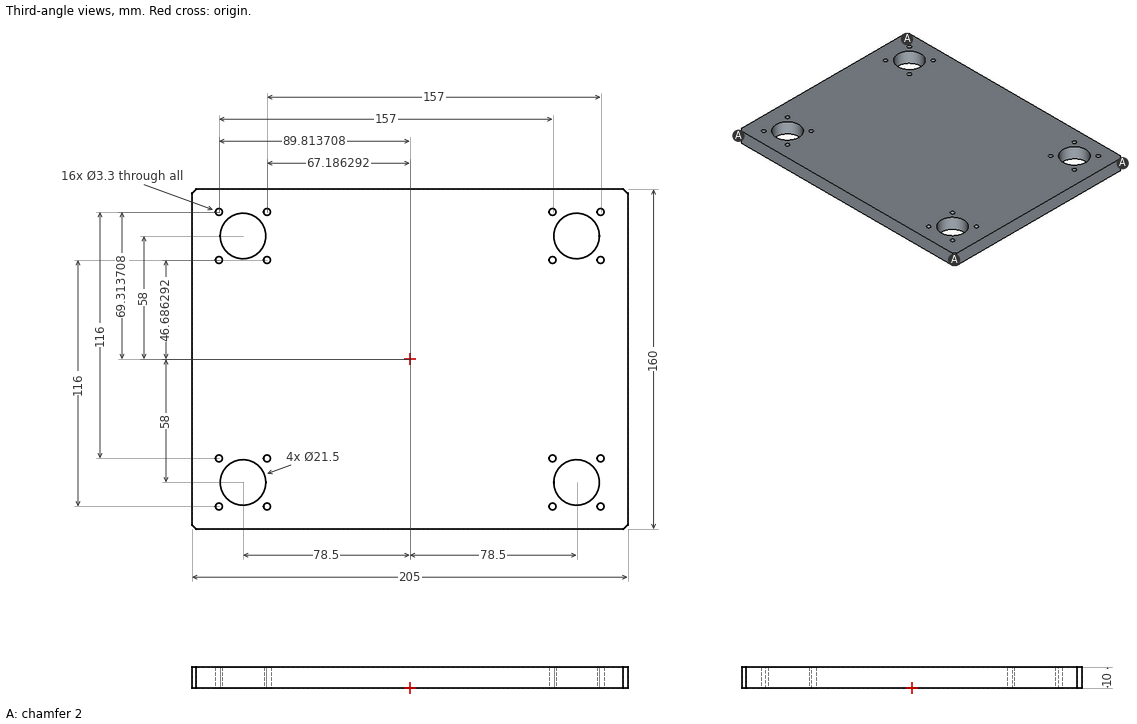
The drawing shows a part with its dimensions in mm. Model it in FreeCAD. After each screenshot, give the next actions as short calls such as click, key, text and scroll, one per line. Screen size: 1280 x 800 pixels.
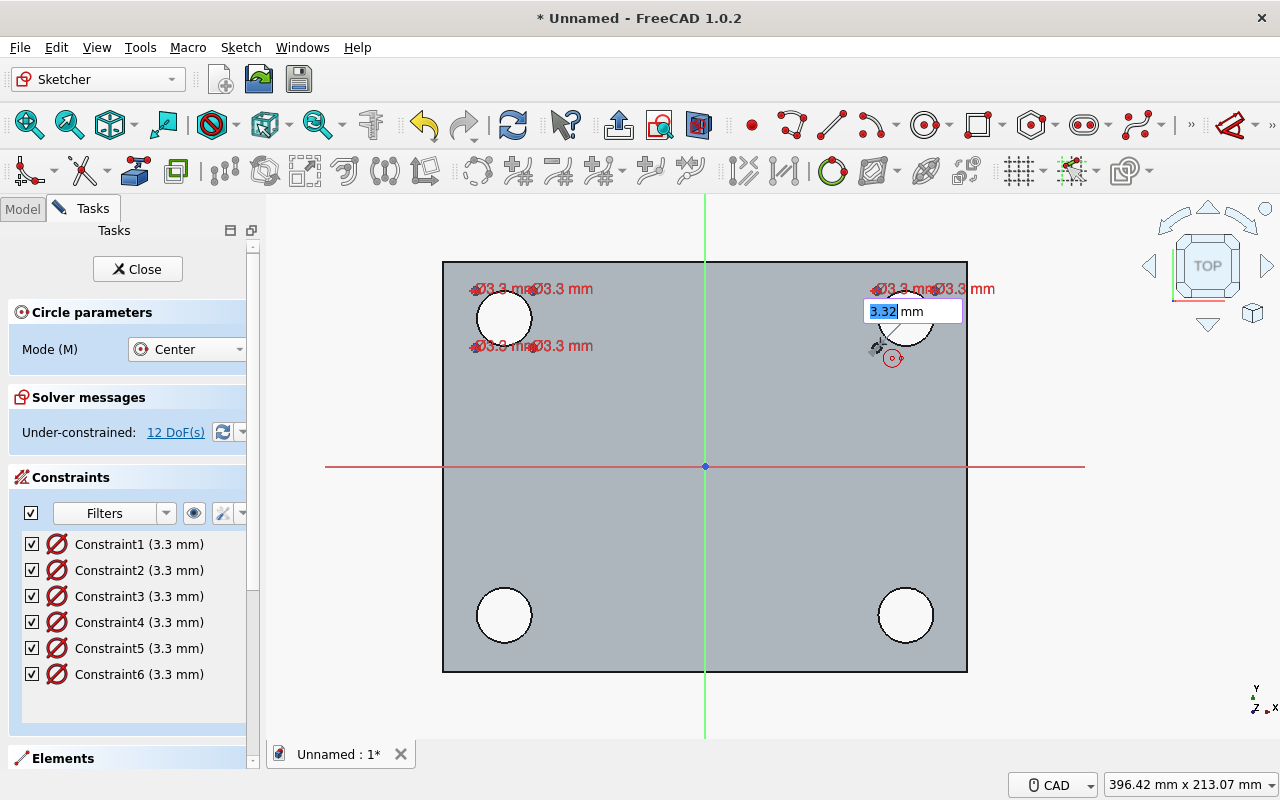
text(3.3)
key(Return)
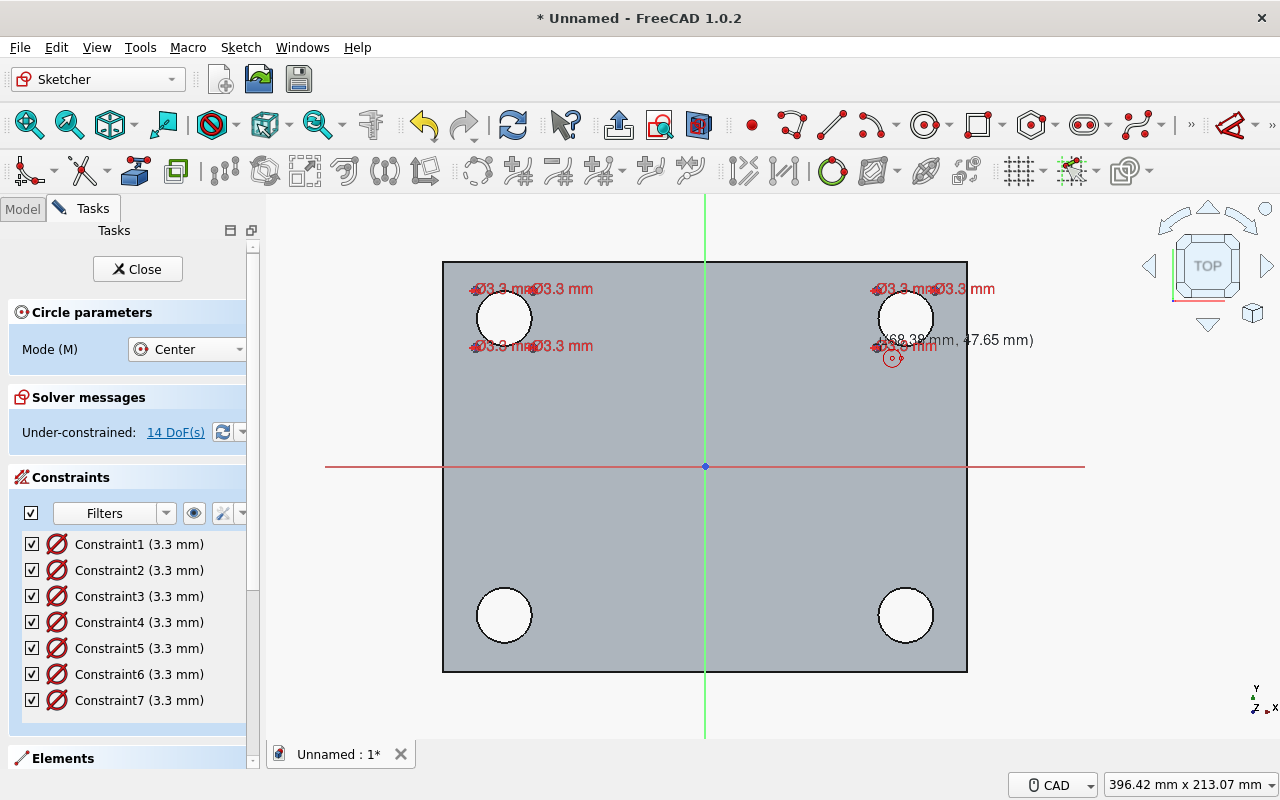
scroll(935, 347, up, 9)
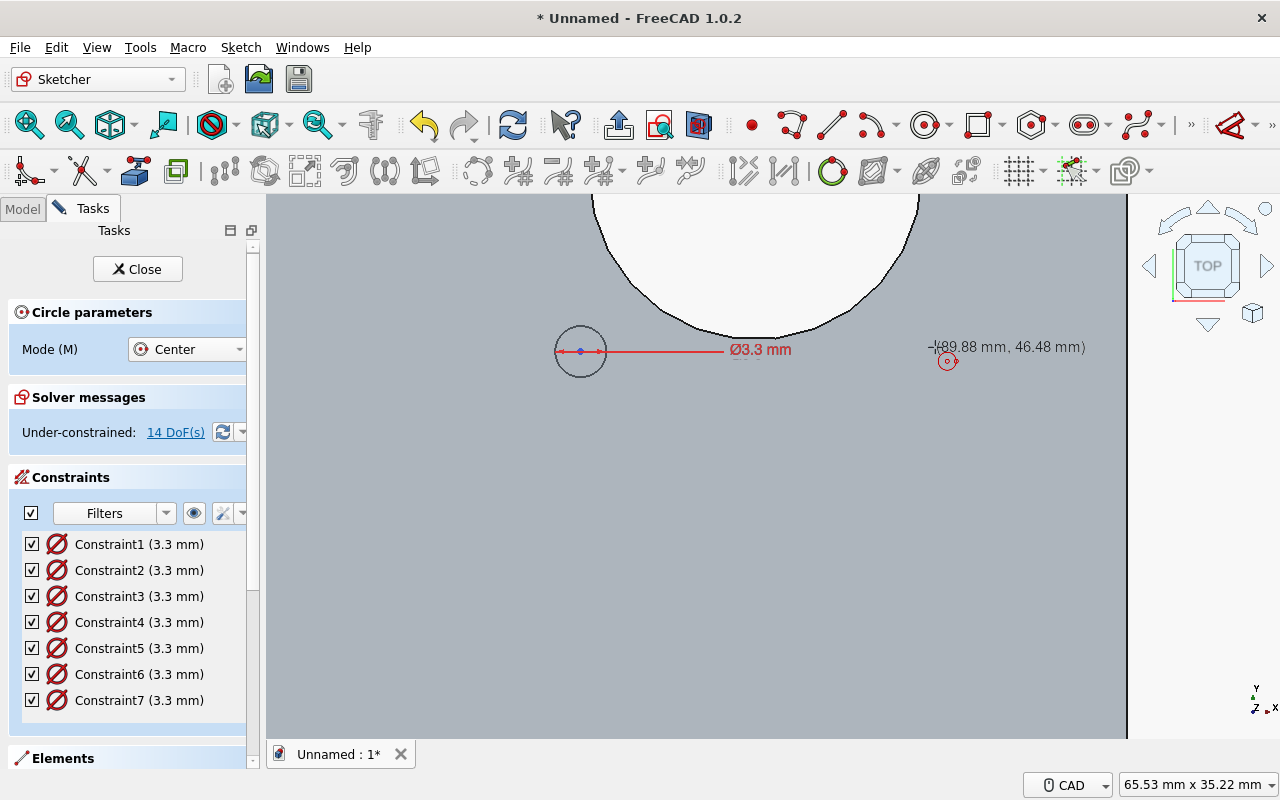
scroll(935, 347, down, 9)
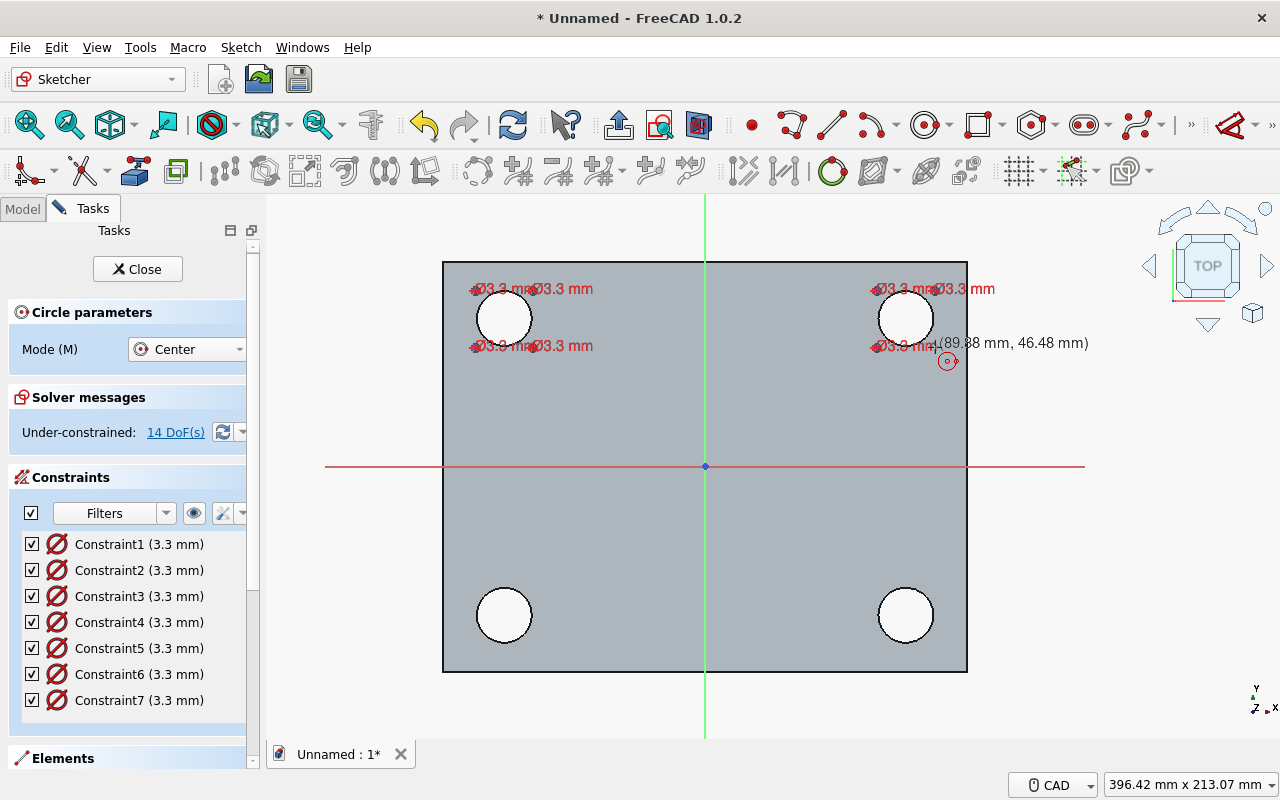
click(935, 347)
move(938, 344)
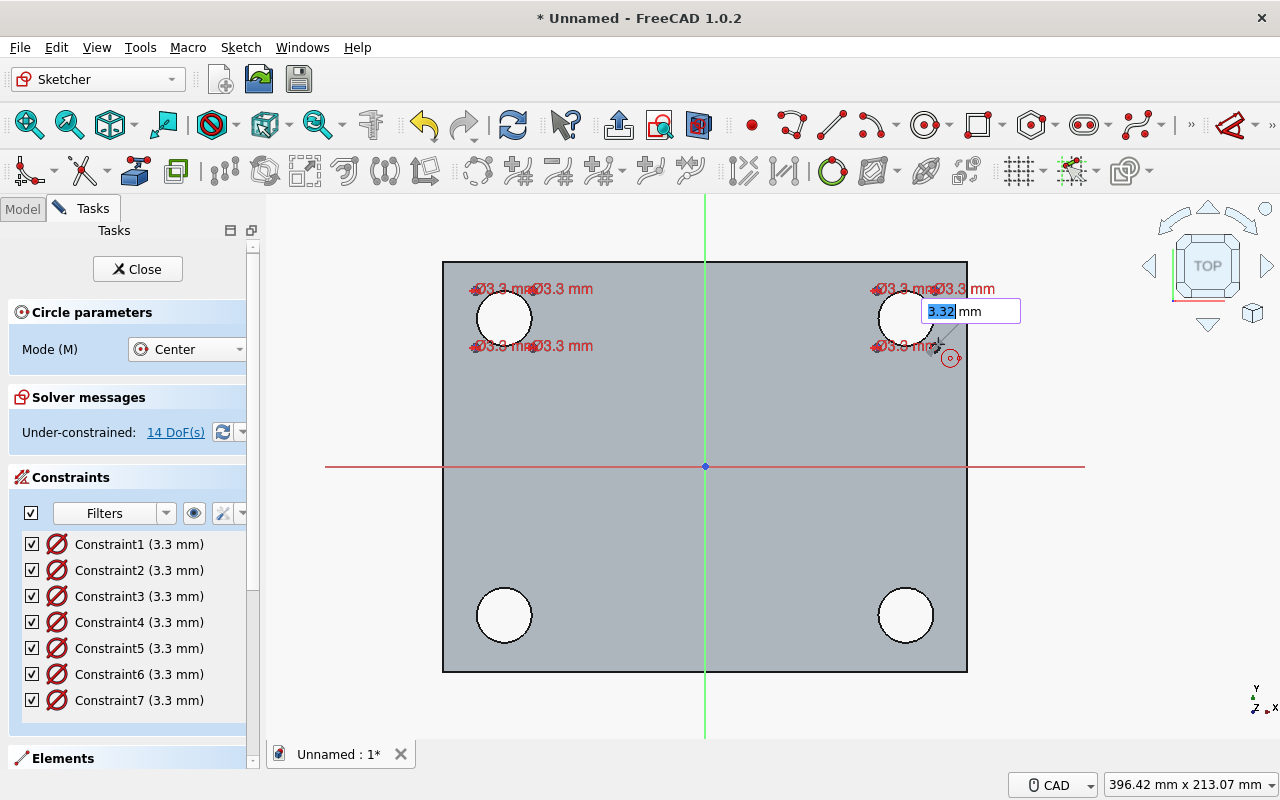
text(3.3)
key(Return)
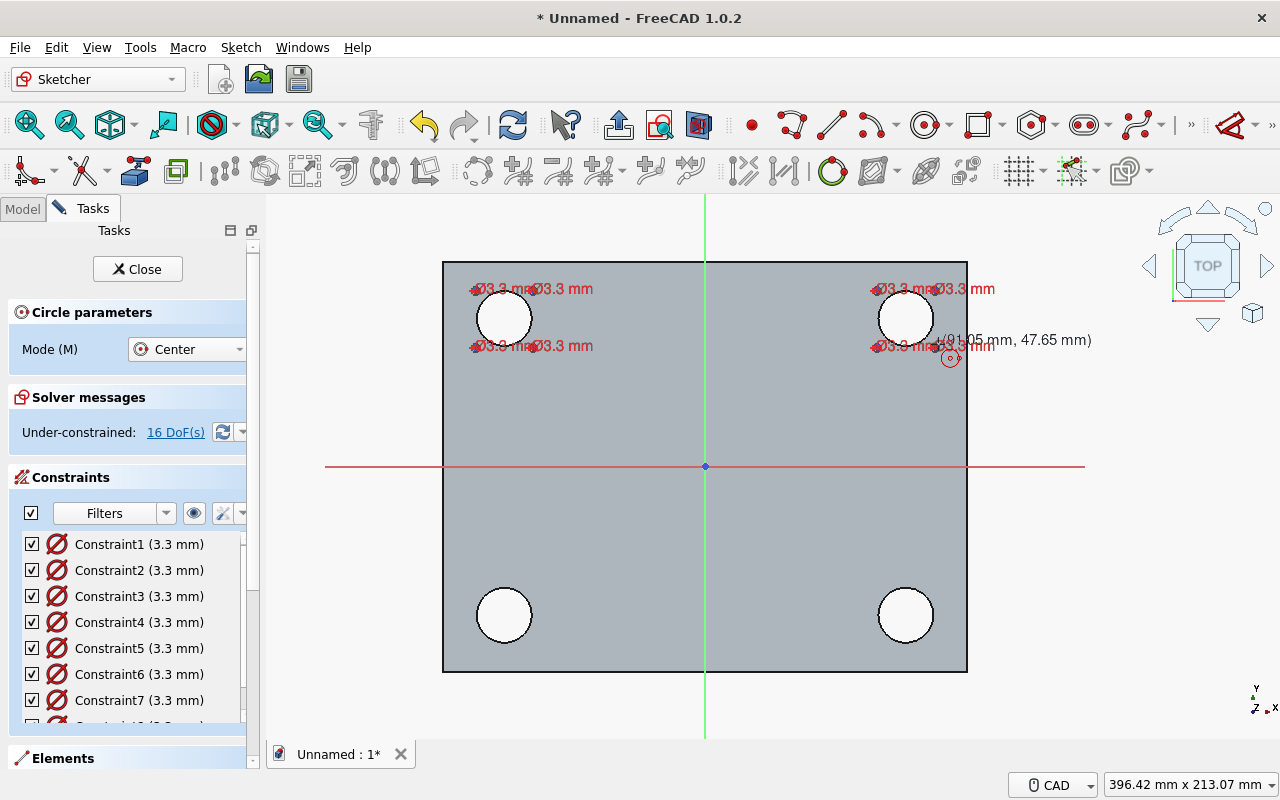
scroll(475, 586, up, 9)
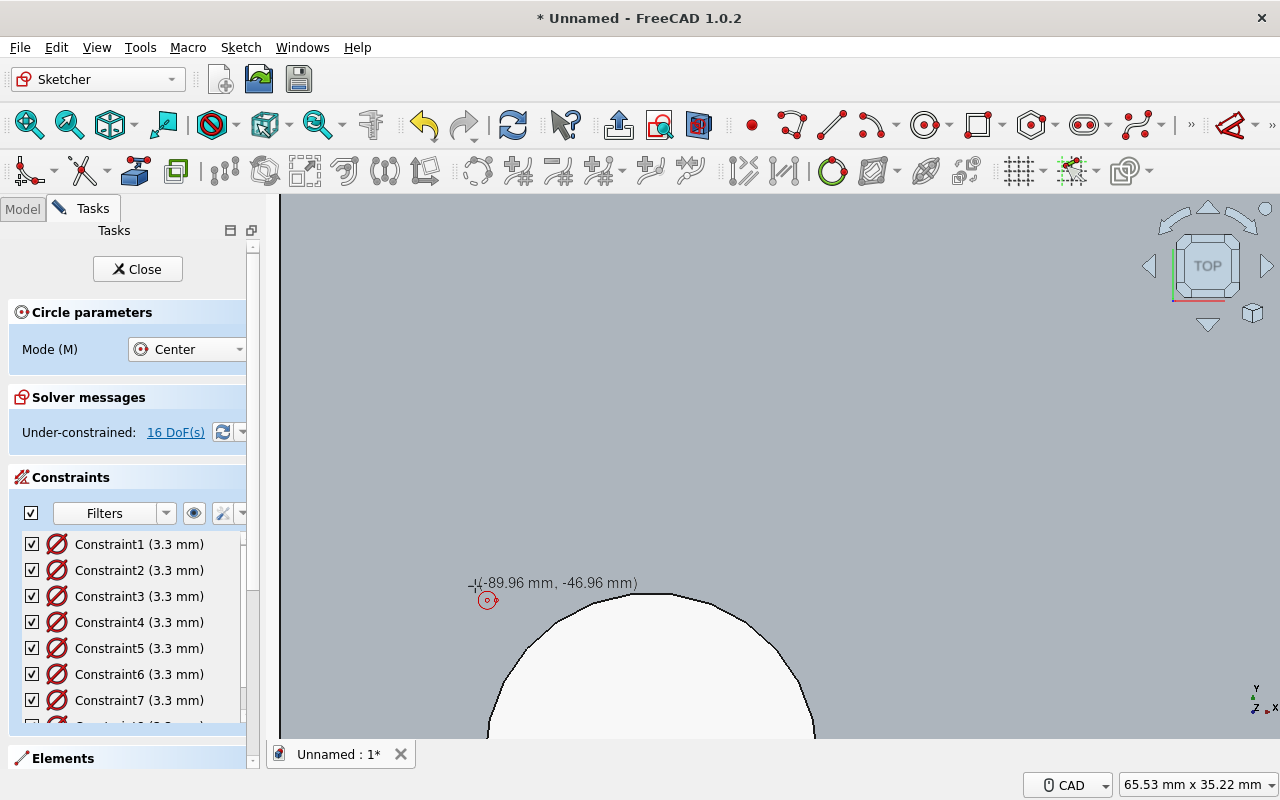
scroll(474, 586, down, 9)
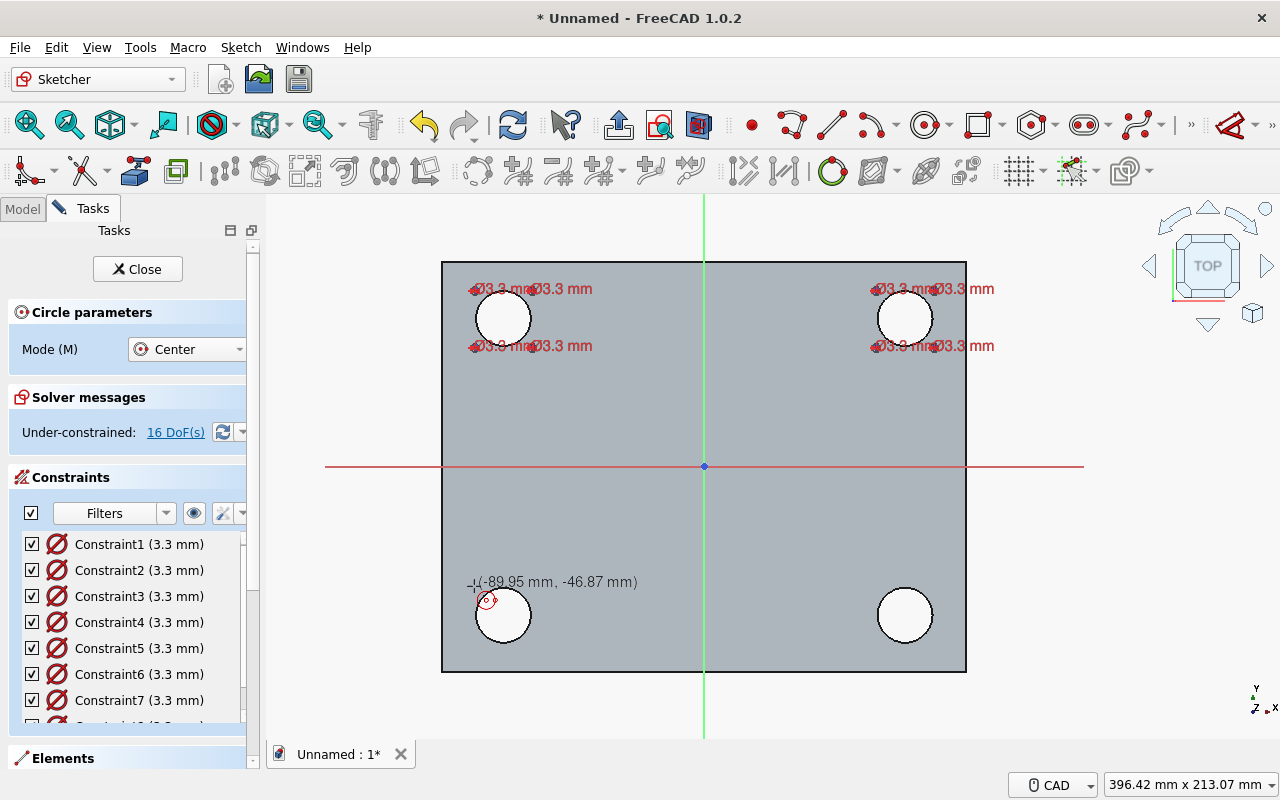
click(475, 586)
move(478, 583)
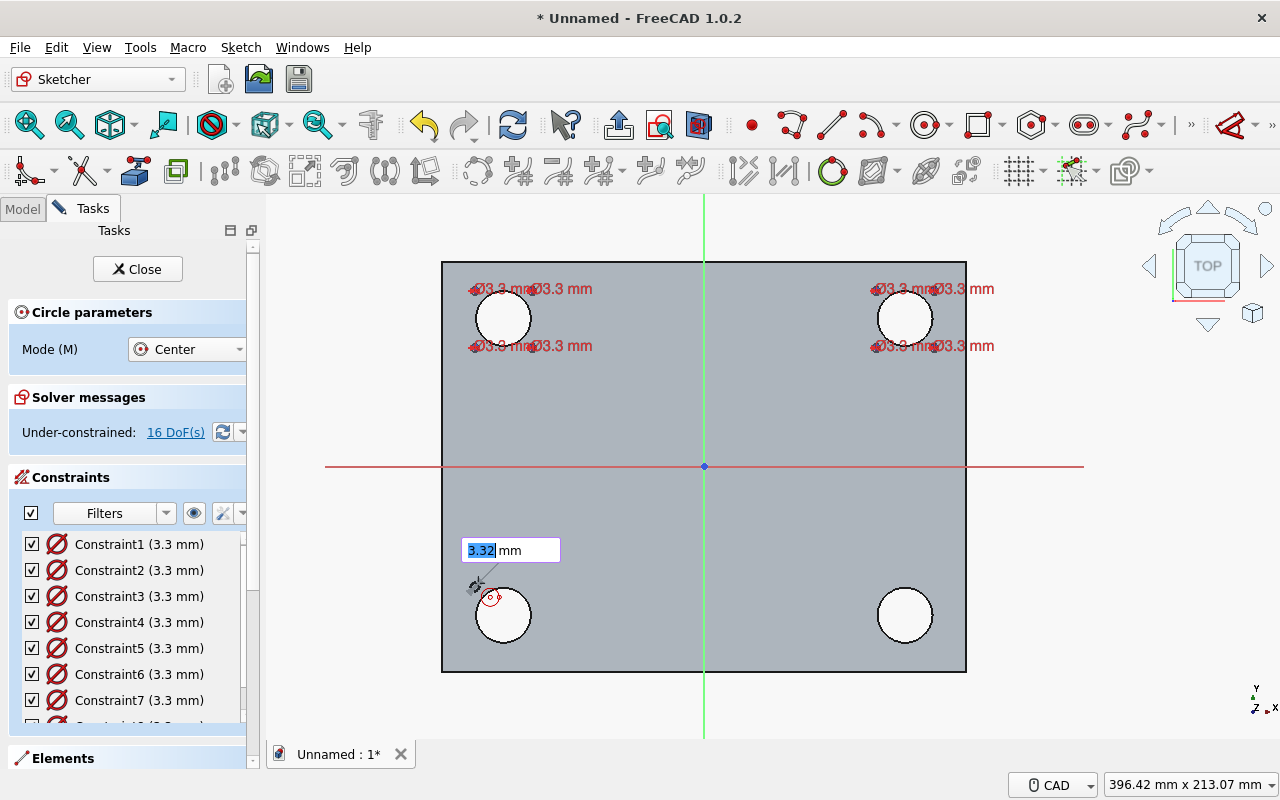
text(3.3)
key(Return)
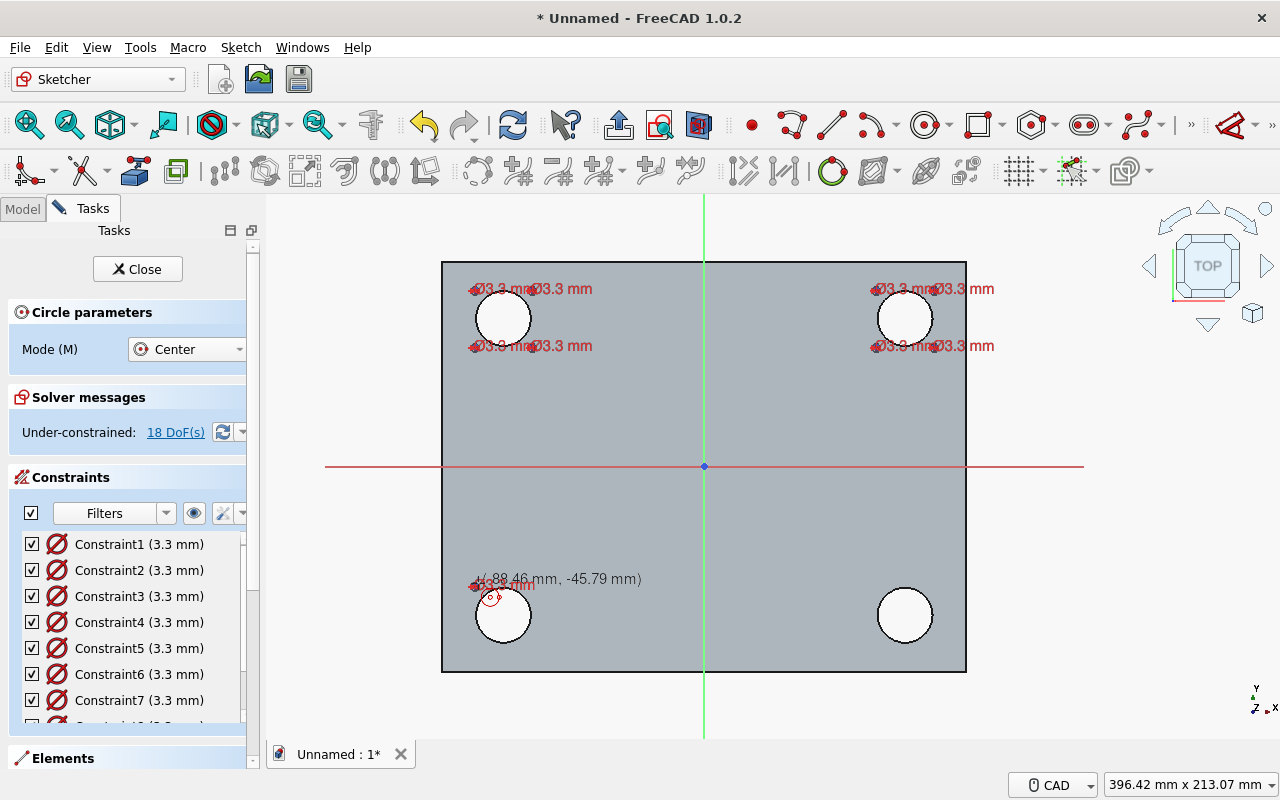
scroll(532, 586, up, 9)